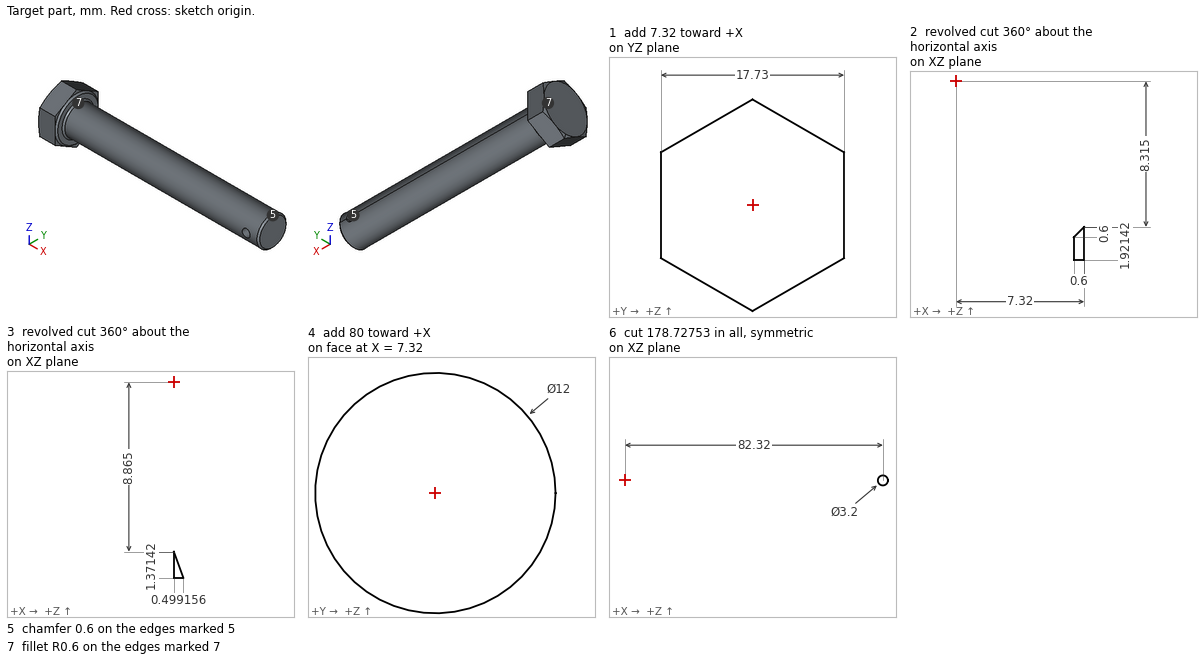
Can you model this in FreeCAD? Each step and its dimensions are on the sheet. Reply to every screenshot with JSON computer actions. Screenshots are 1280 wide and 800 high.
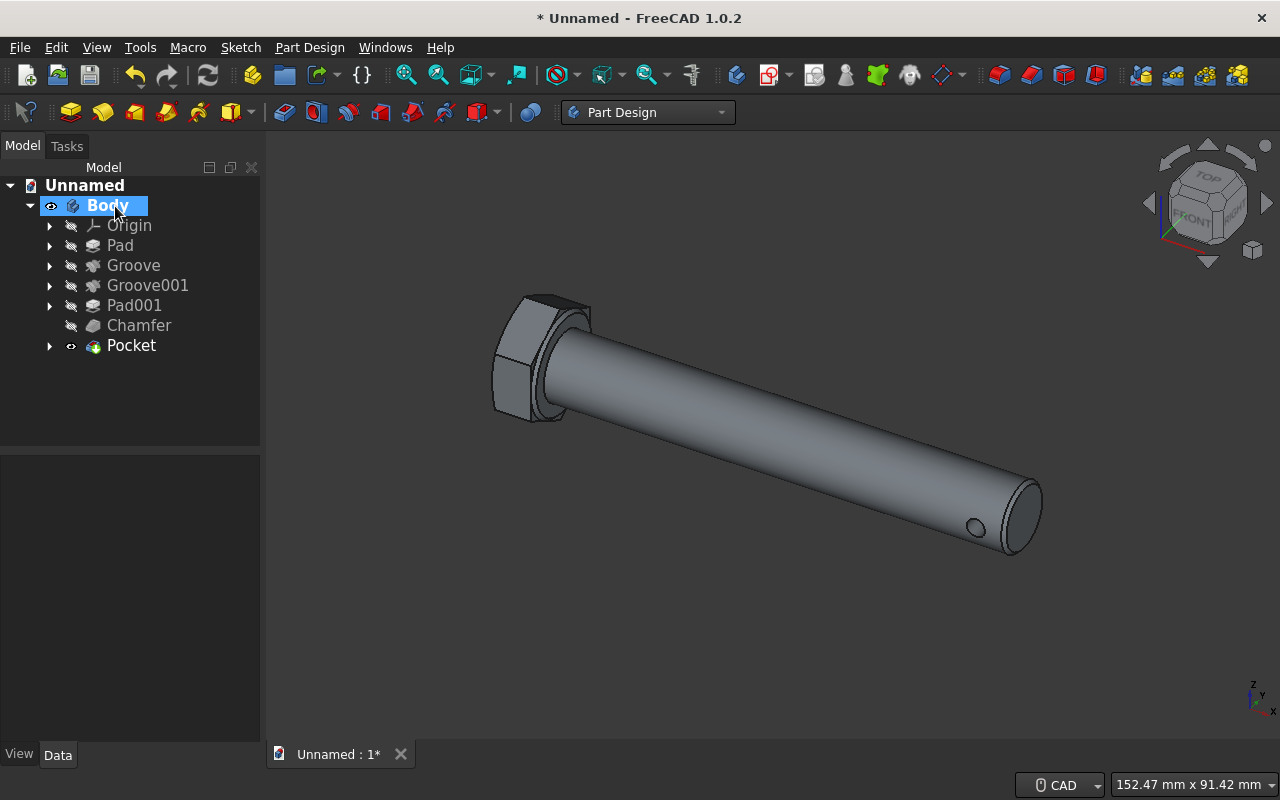
{"action": "key", "text": "0"}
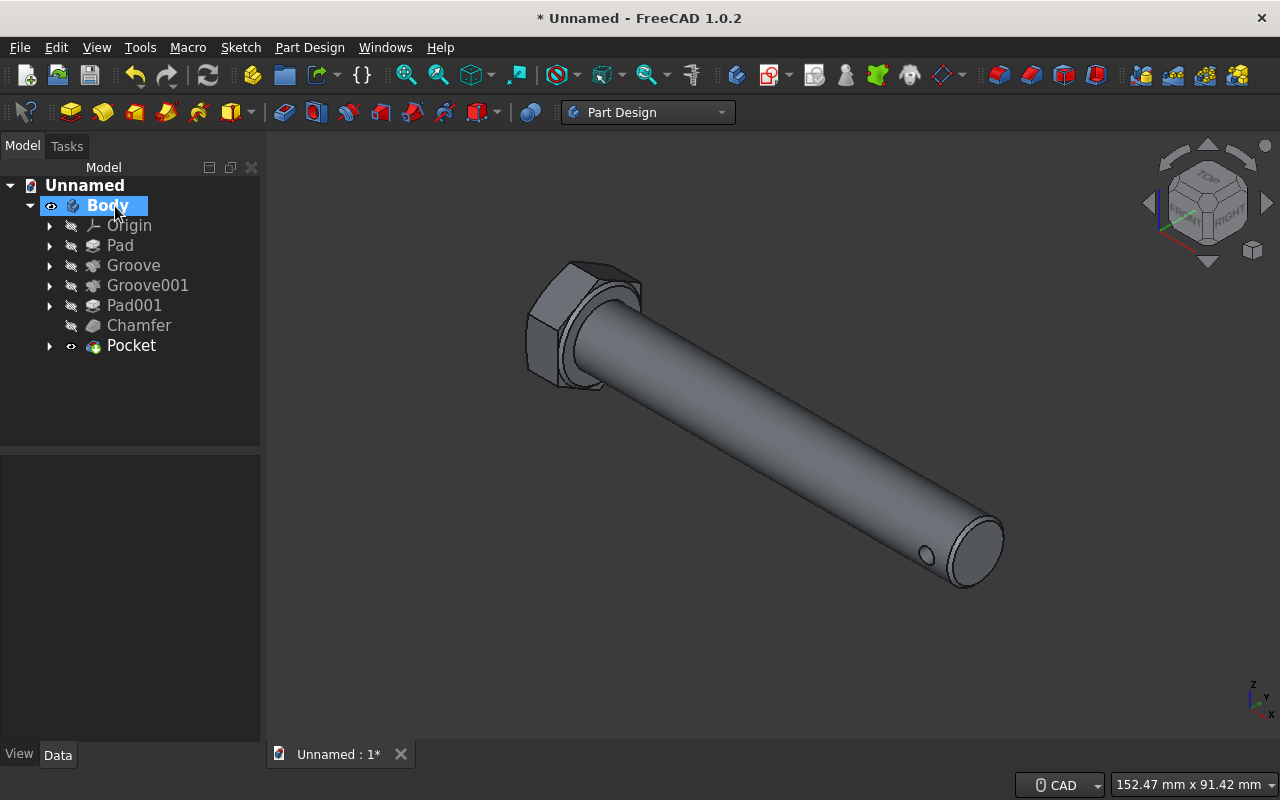
{"action": "key", "text": "2"}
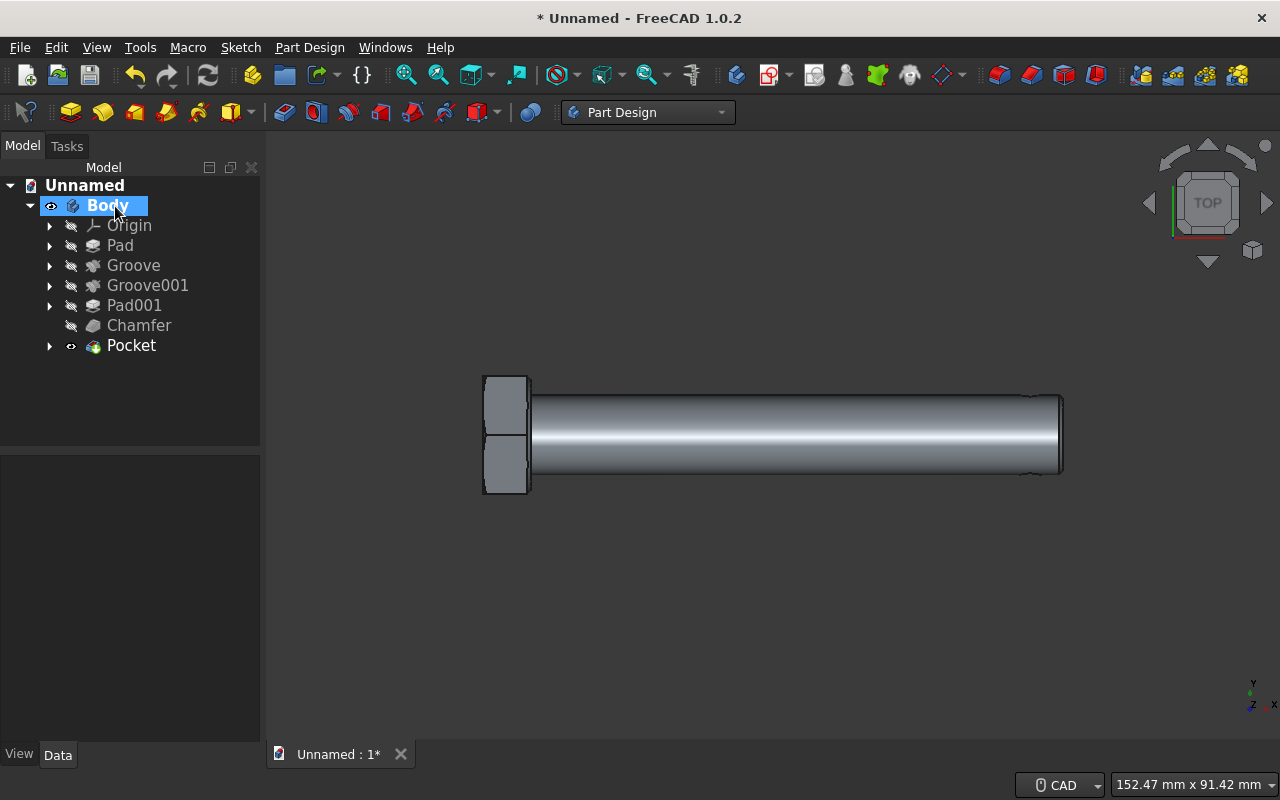
{"action": "key", "text": "1"}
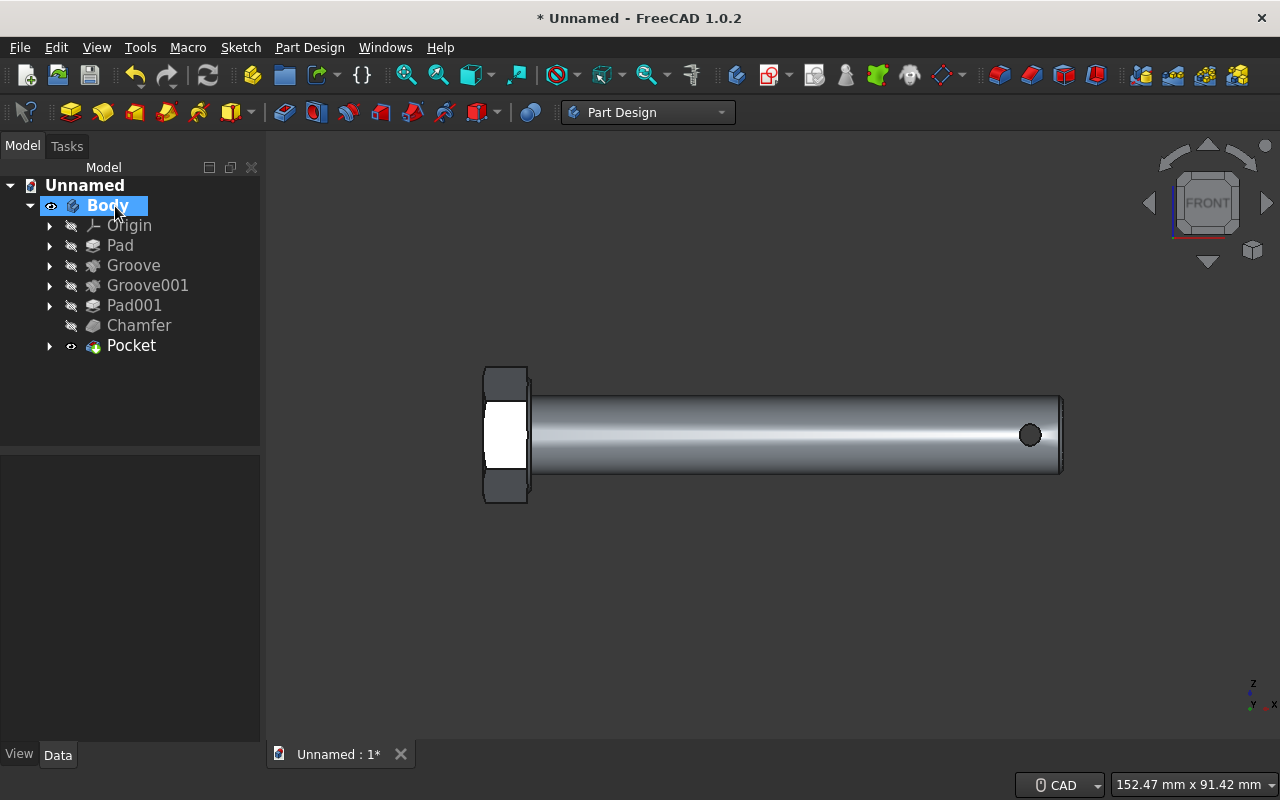
{"action": "key", "text": "3"}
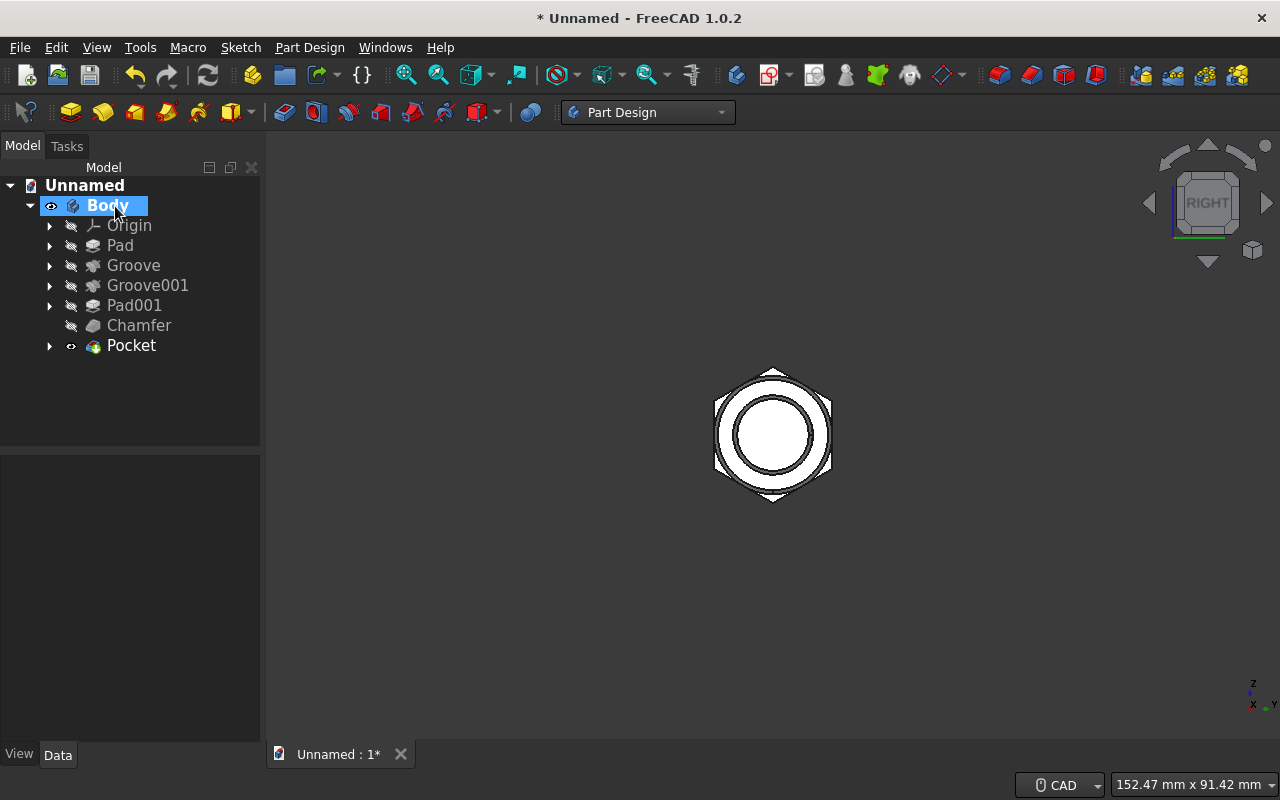
{"action": "left_click", "coordinate": [408, 76]}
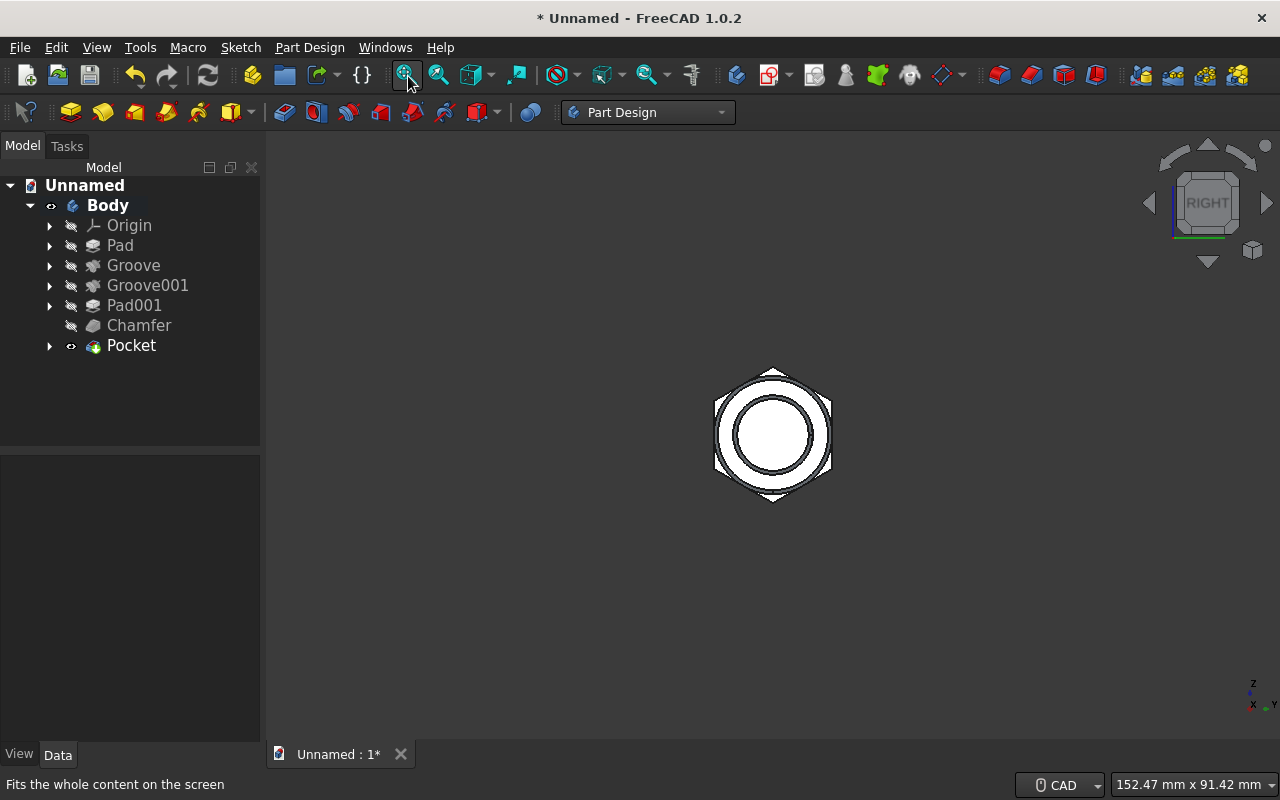
{"action": "key", "text": "5"}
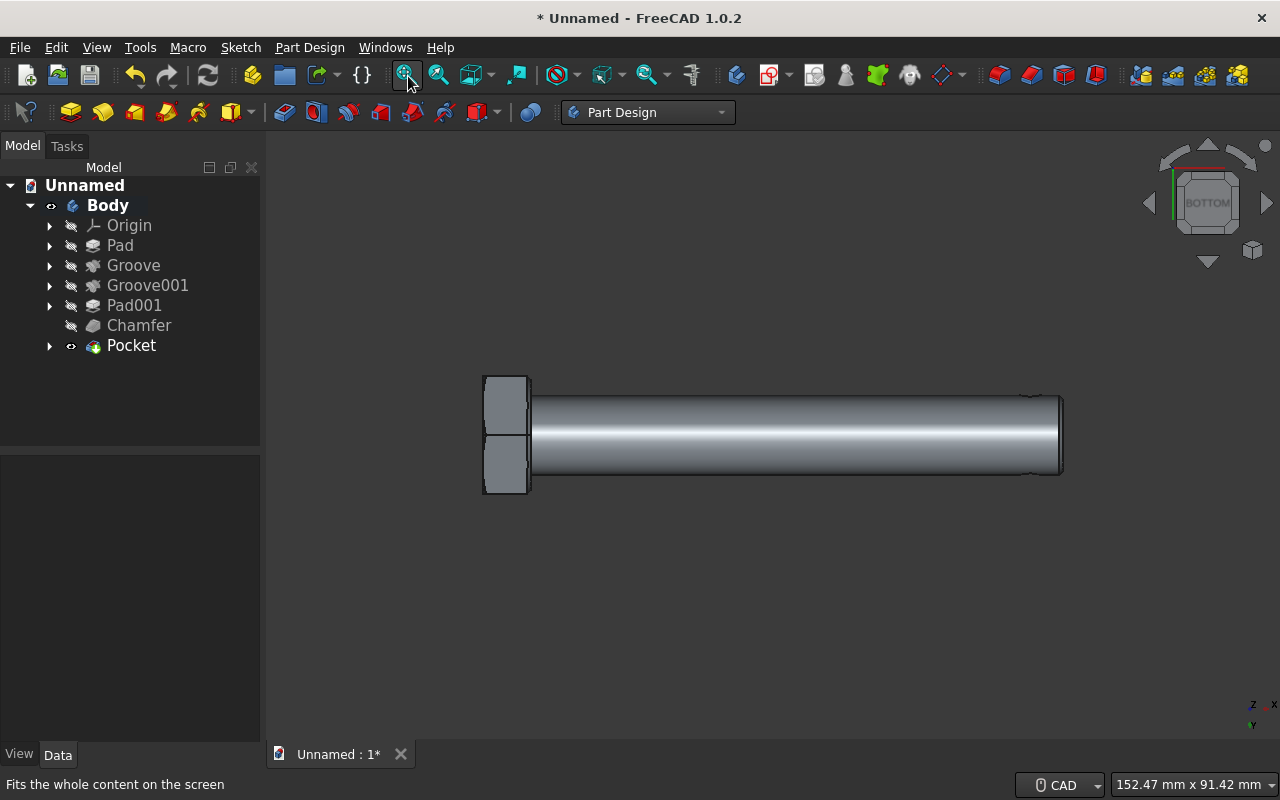
{"action": "key", "text": "4"}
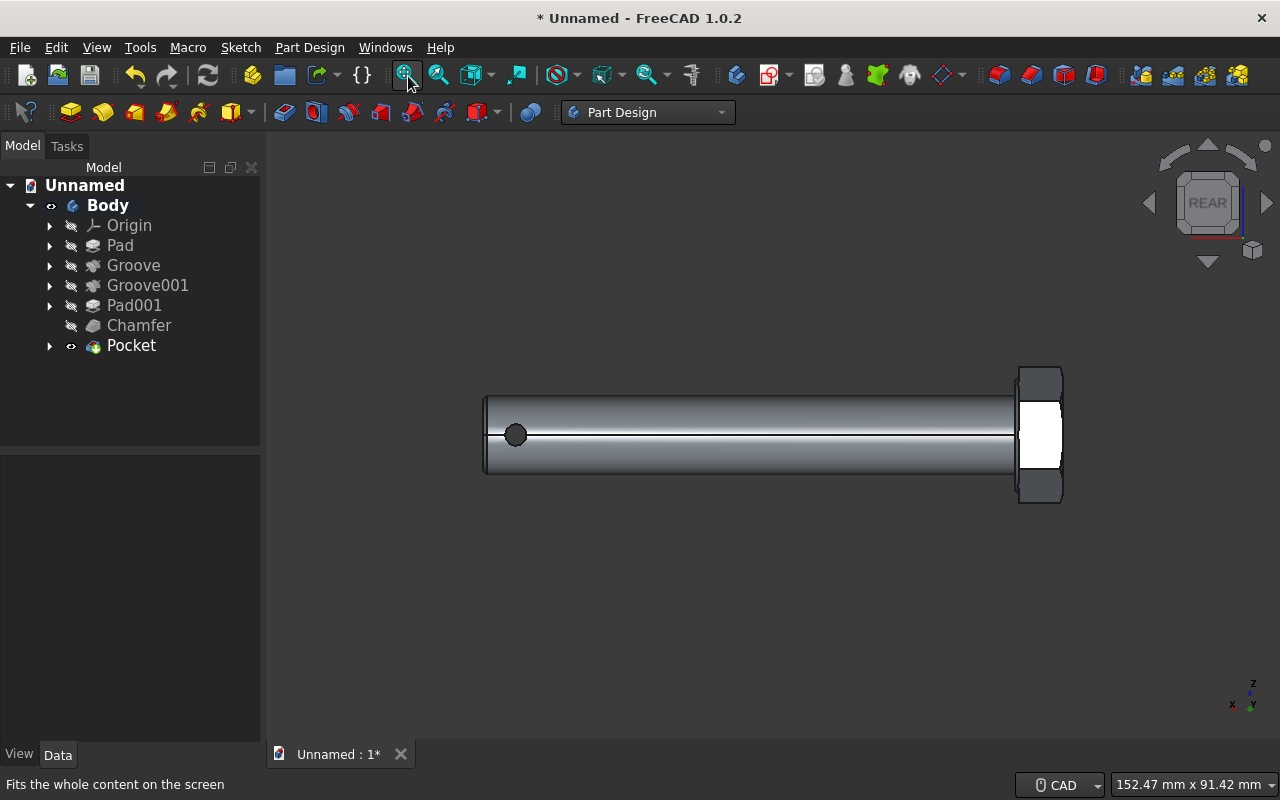
{"action": "key", "text": "6"}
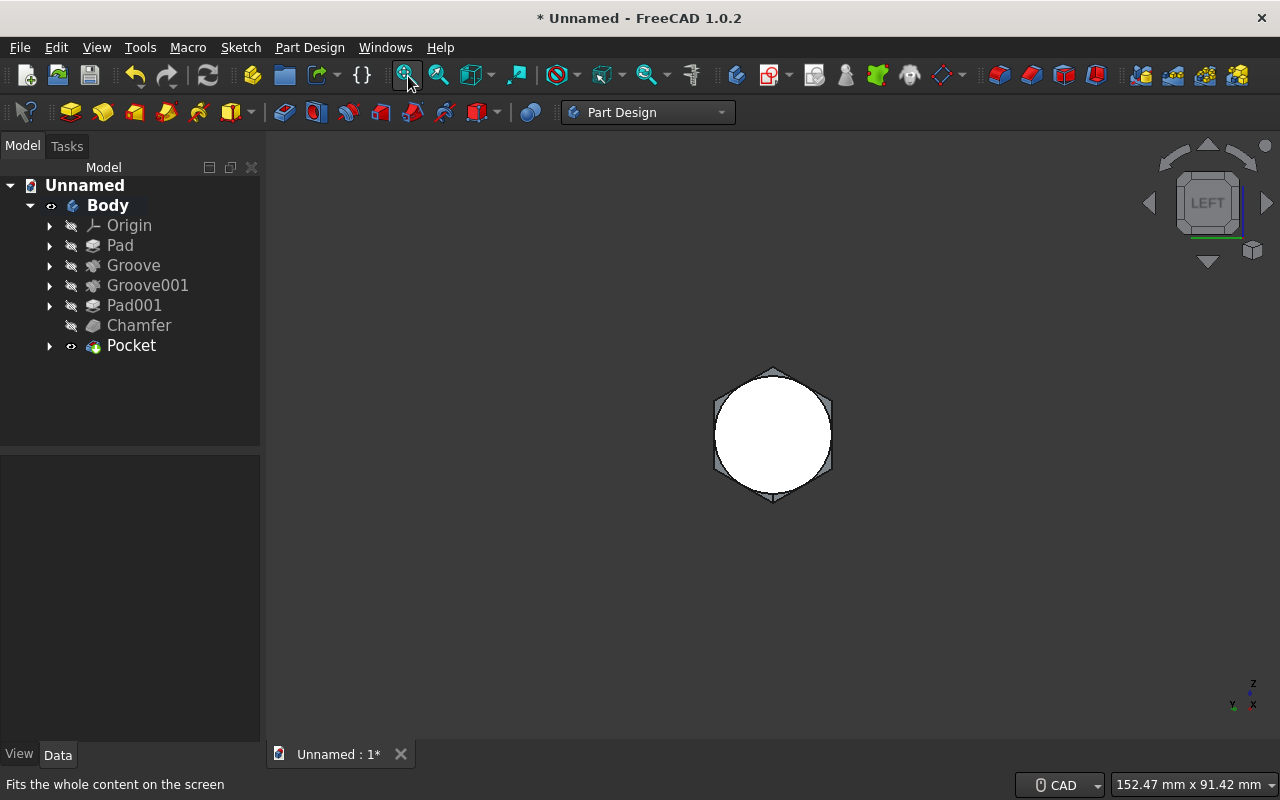
{"action": "left_click", "coordinate": [408, 76]}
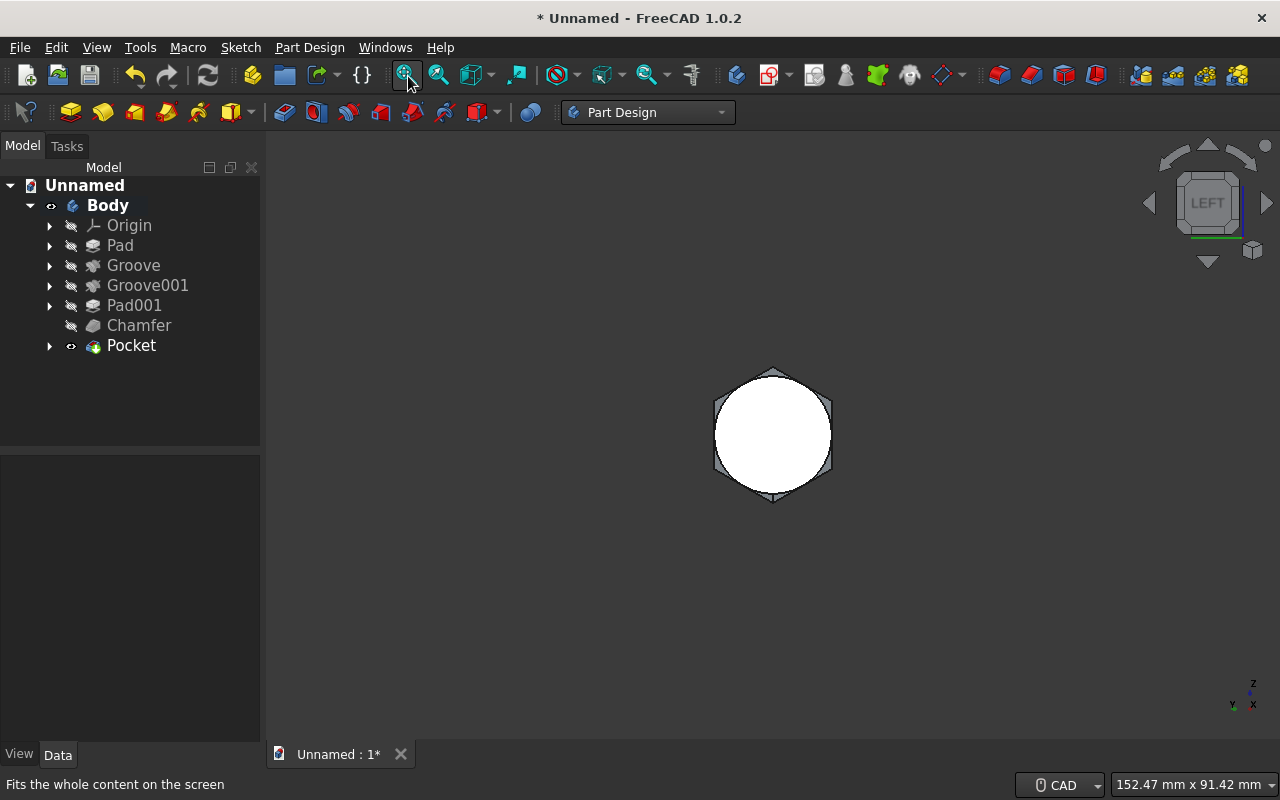
{"action": "key", "text": "v 3"}